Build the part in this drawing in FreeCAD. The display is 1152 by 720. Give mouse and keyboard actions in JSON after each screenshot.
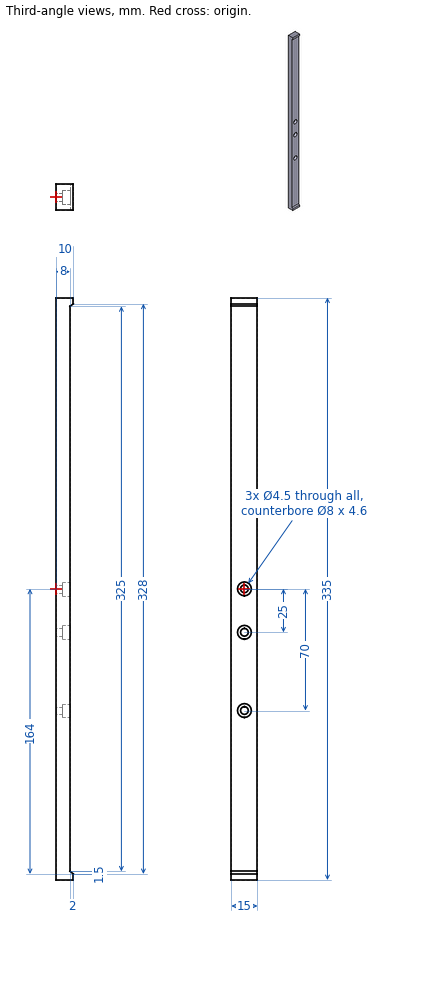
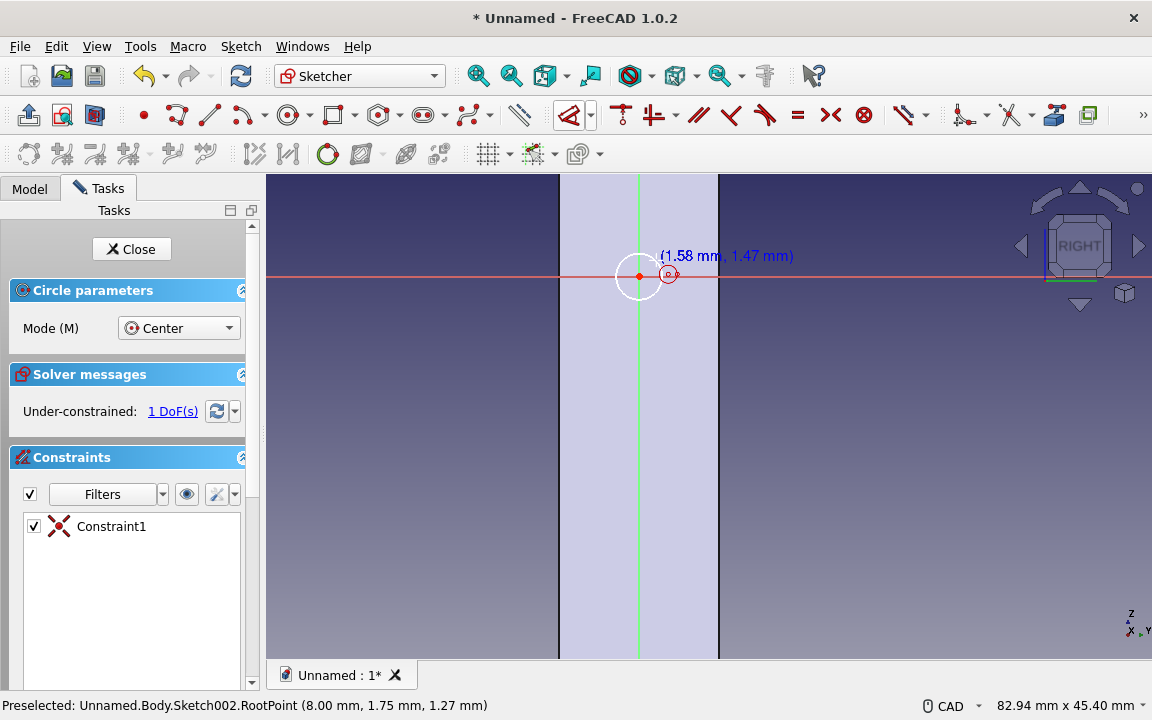
{"action": "scroll", "coordinate": [641, 280], "scroll_direction": "down", "scroll_amount": 5}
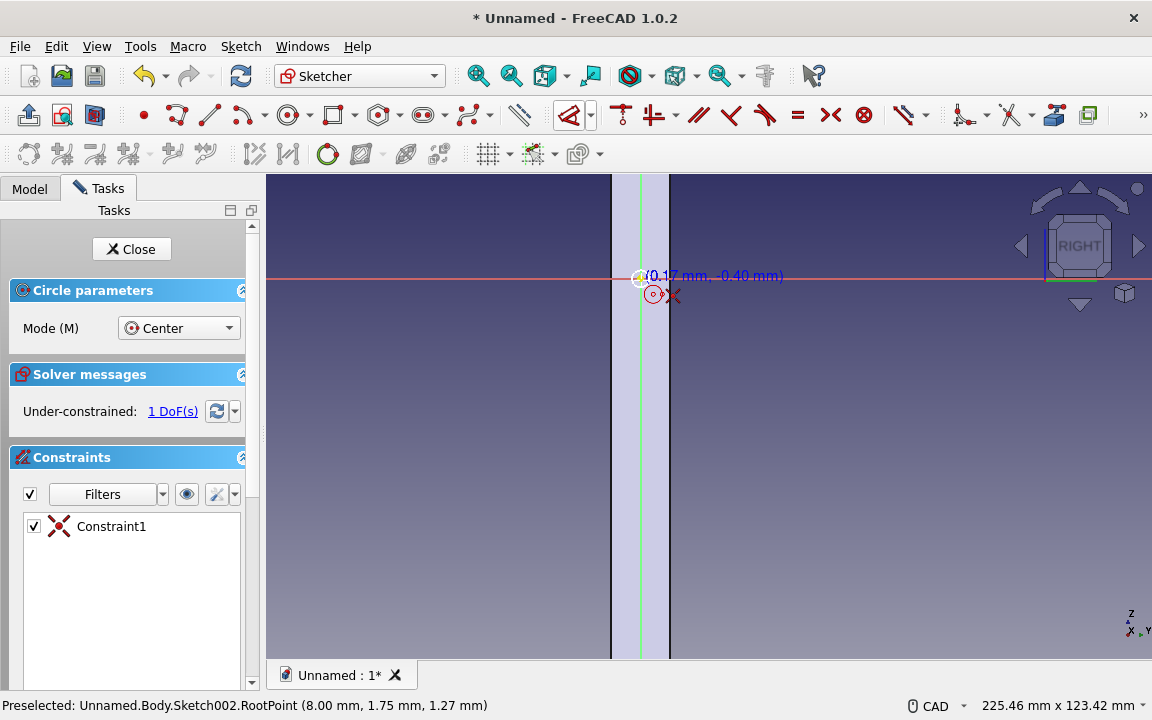
{"action": "scroll", "coordinate": [641, 554], "scroll_direction": "up", "scroll_amount": 5}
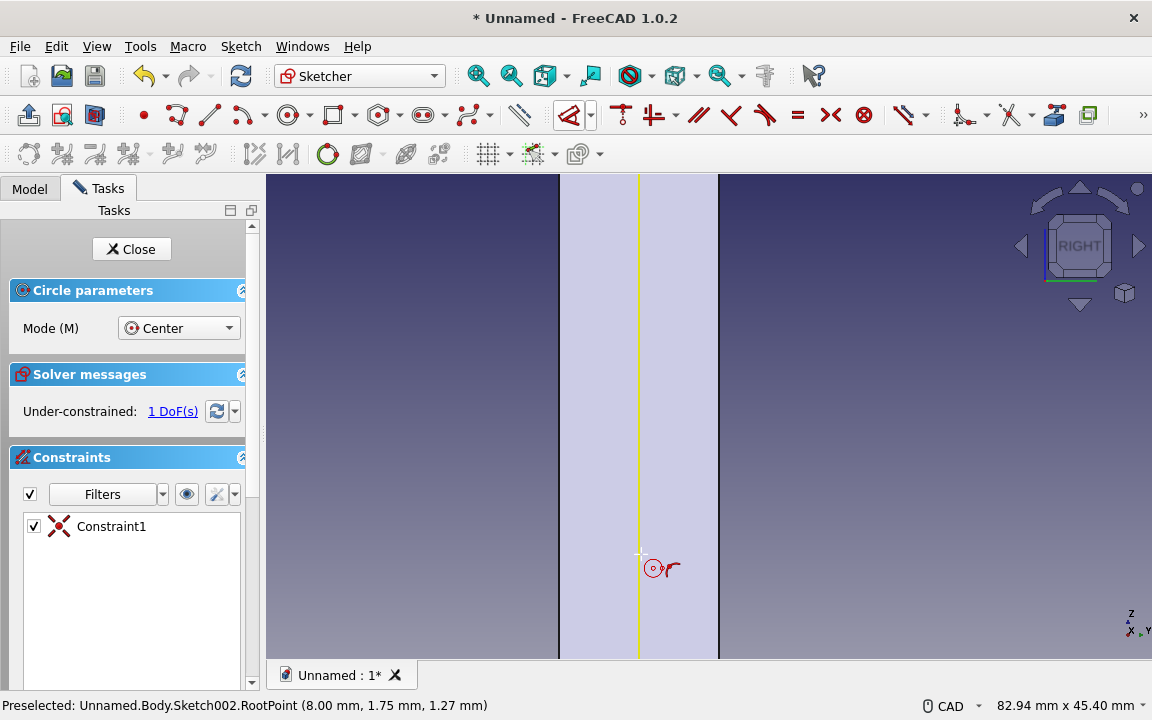
{"action": "left_click", "coordinate": [639, 553]}
{"action": "left_click", "coordinate": [656, 536]}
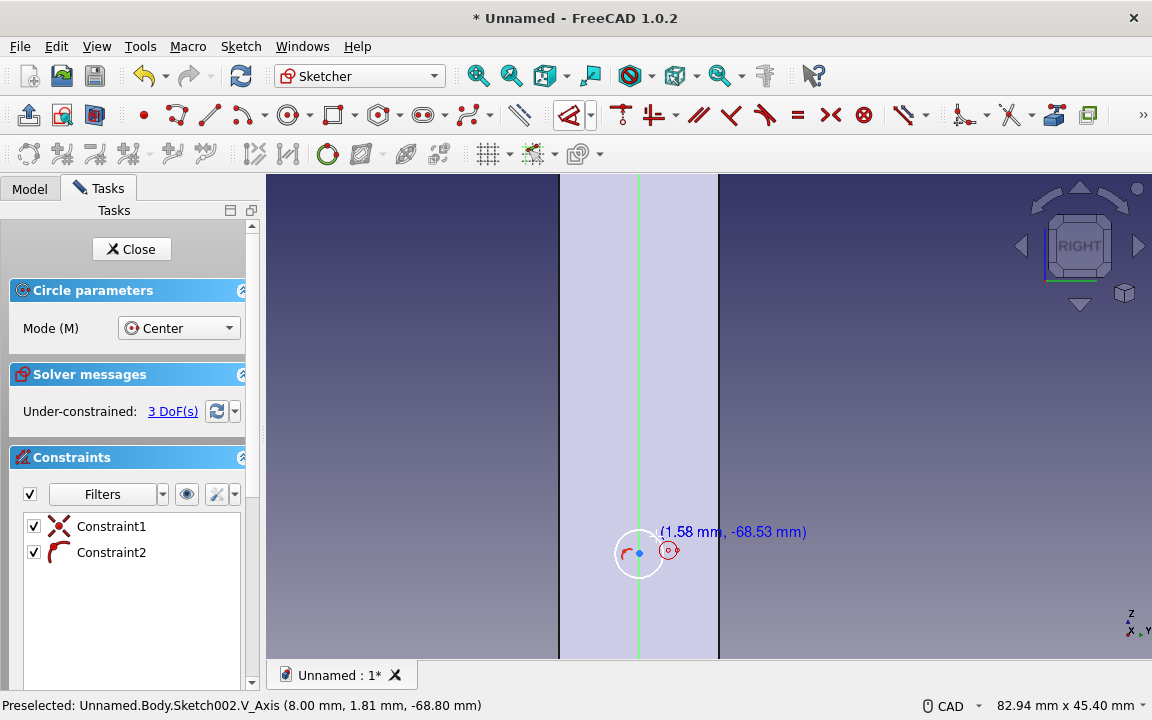
{"action": "scroll", "coordinate": [641, 555], "scroll_direction": "down", "scroll_amount": 5}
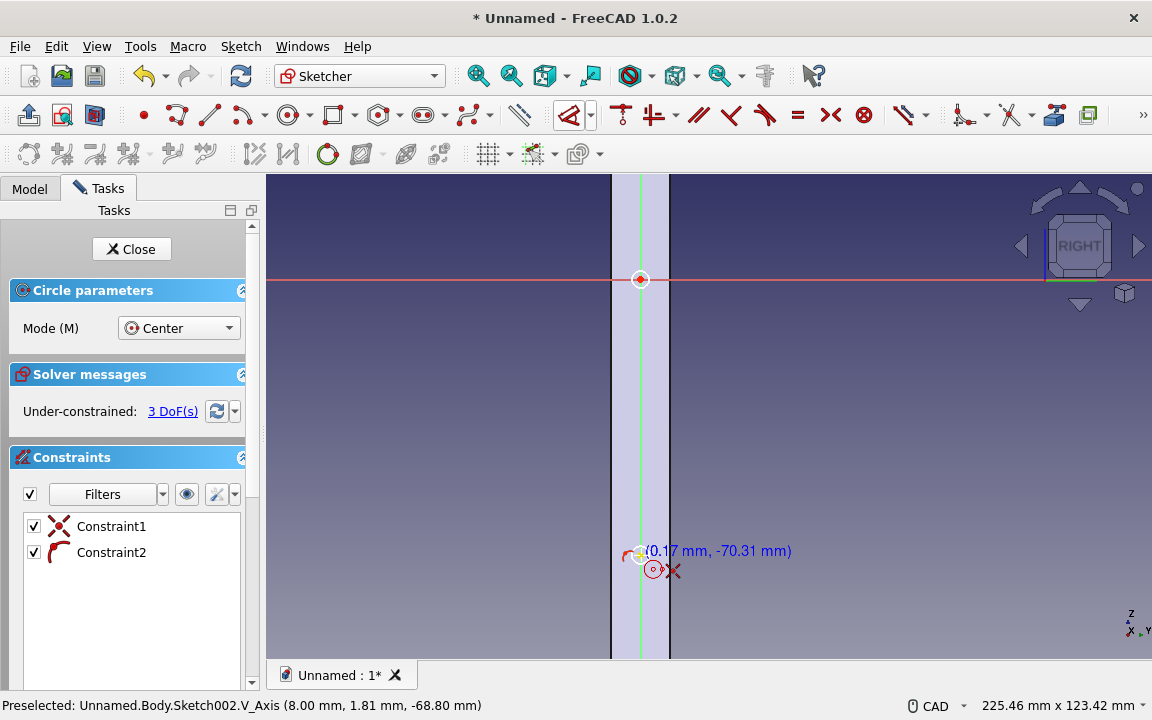
{"action": "scroll", "coordinate": [641, 378], "scroll_direction": "up", "scroll_amount": 5}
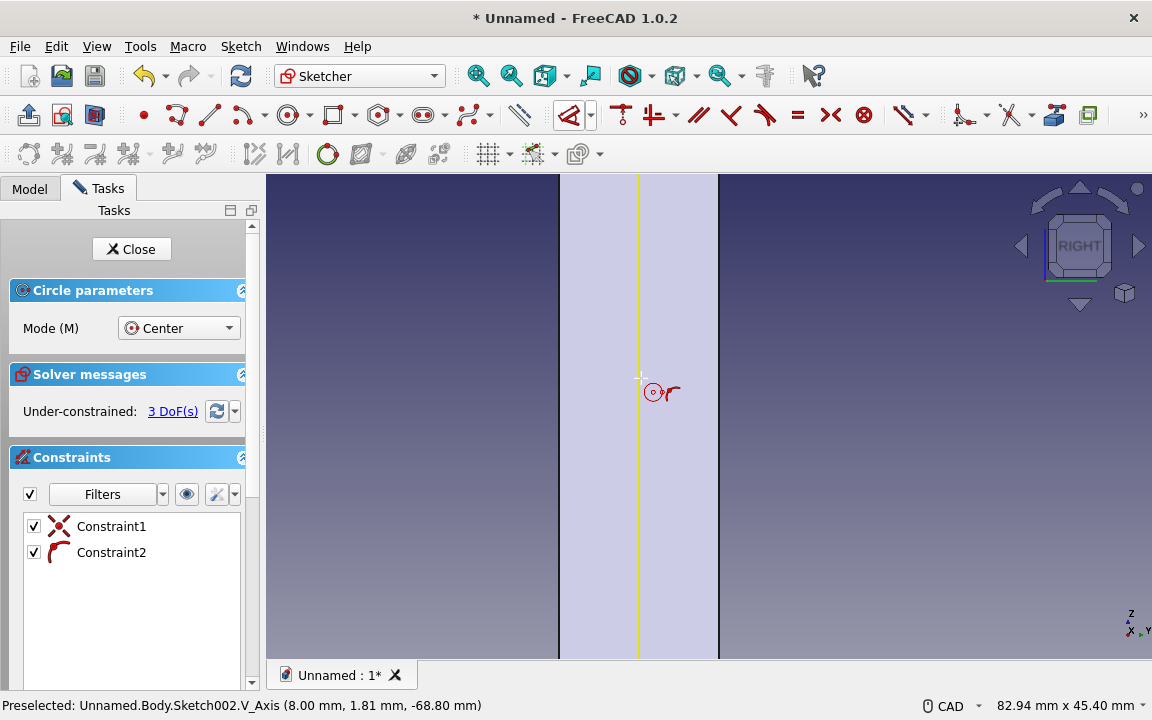
{"action": "left_click", "coordinate": [639, 377]}
{"action": "left_click", "coordinate": [656, 360]}
{"action": "key", "text": "Escape"}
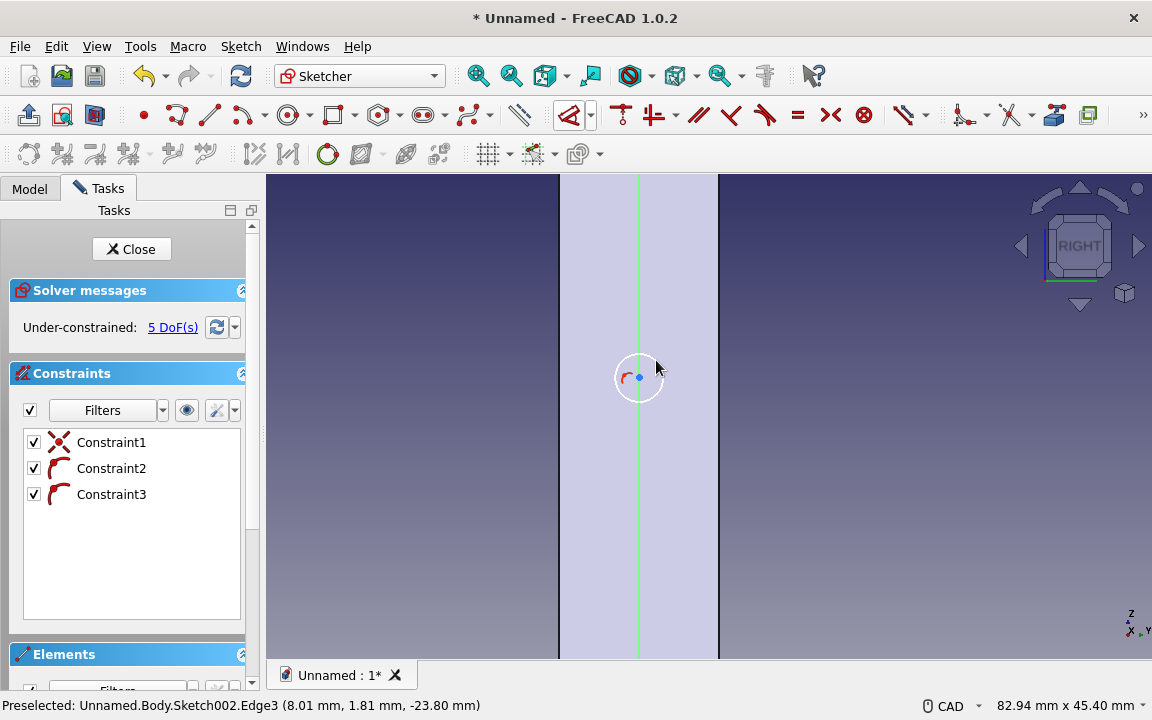
{"action": "scroll", "coordinate": [641, 377], "scroll_direction": "down", "scroll_amount": 5}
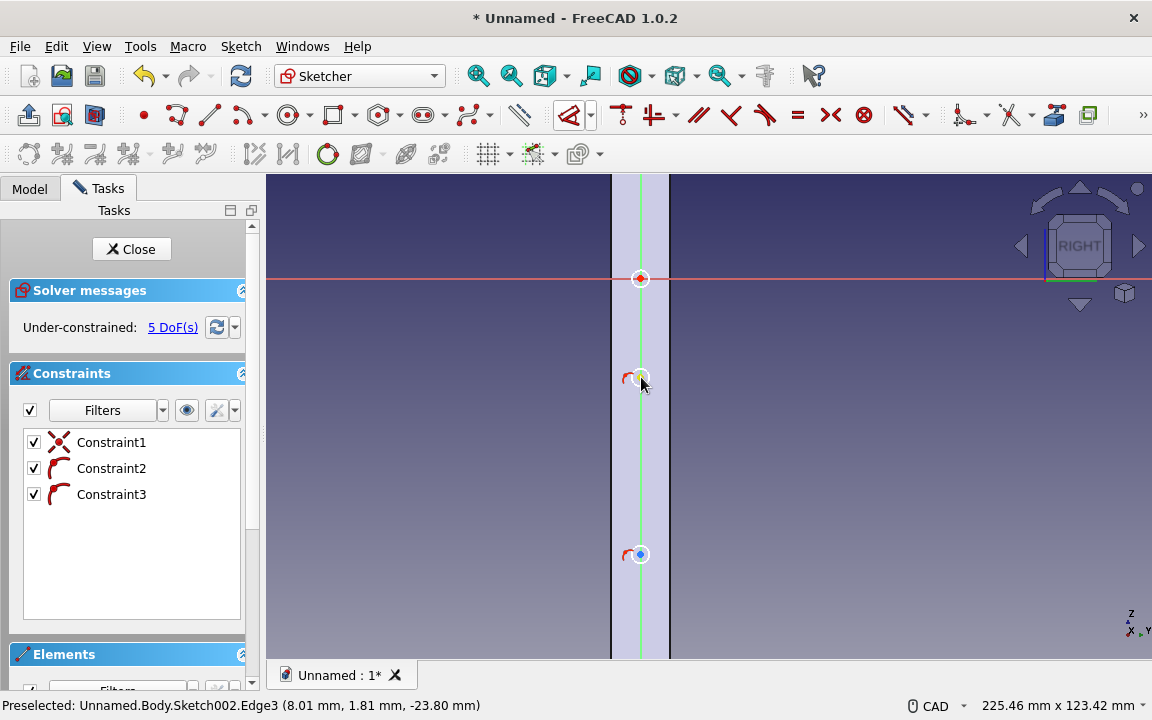
{"action": "scroll", "coordinate": [647, 273], "scroll_direction": "up", "scroll_amount": 5}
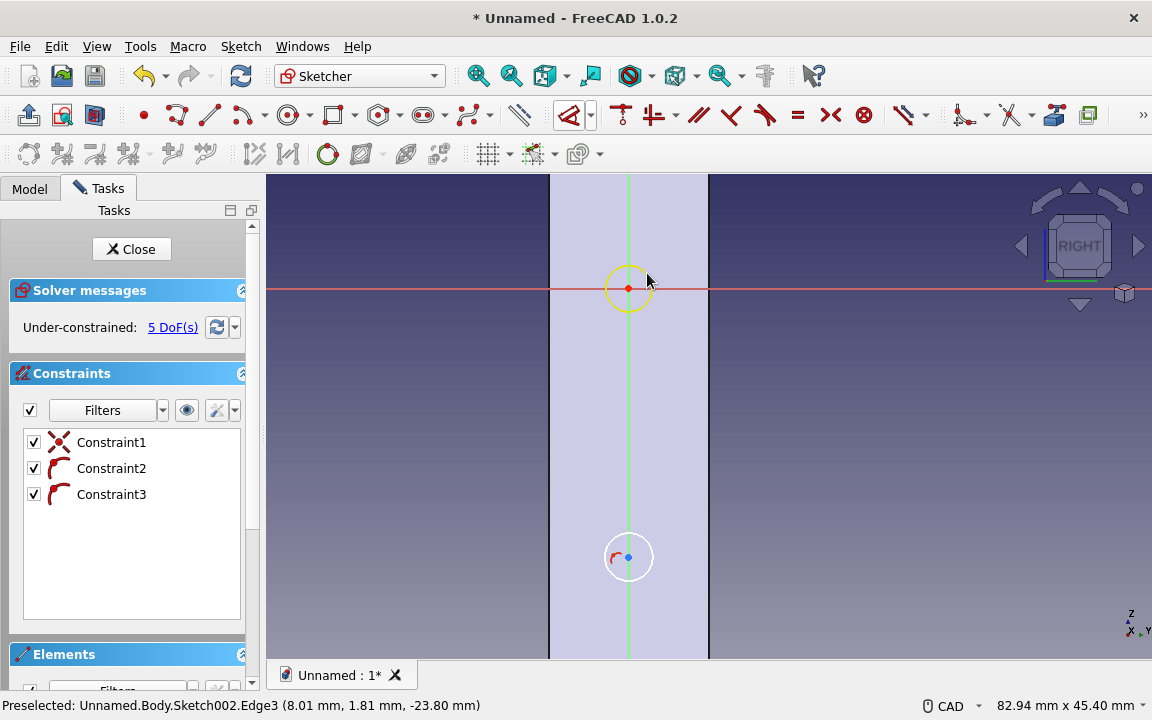
{"action": "left_click", "coordinate": [645, 272]}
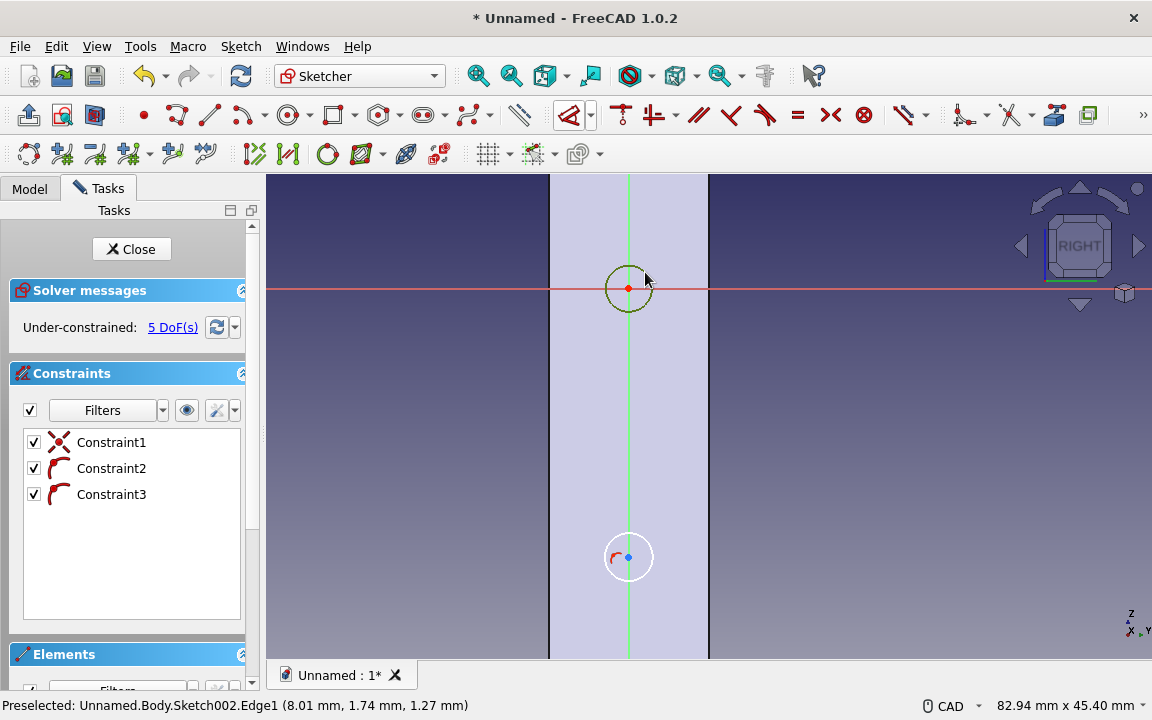
{"action": "scroll", "coordinate": [647, 273], "scroll_direction": "down", "scroll_amount": 5}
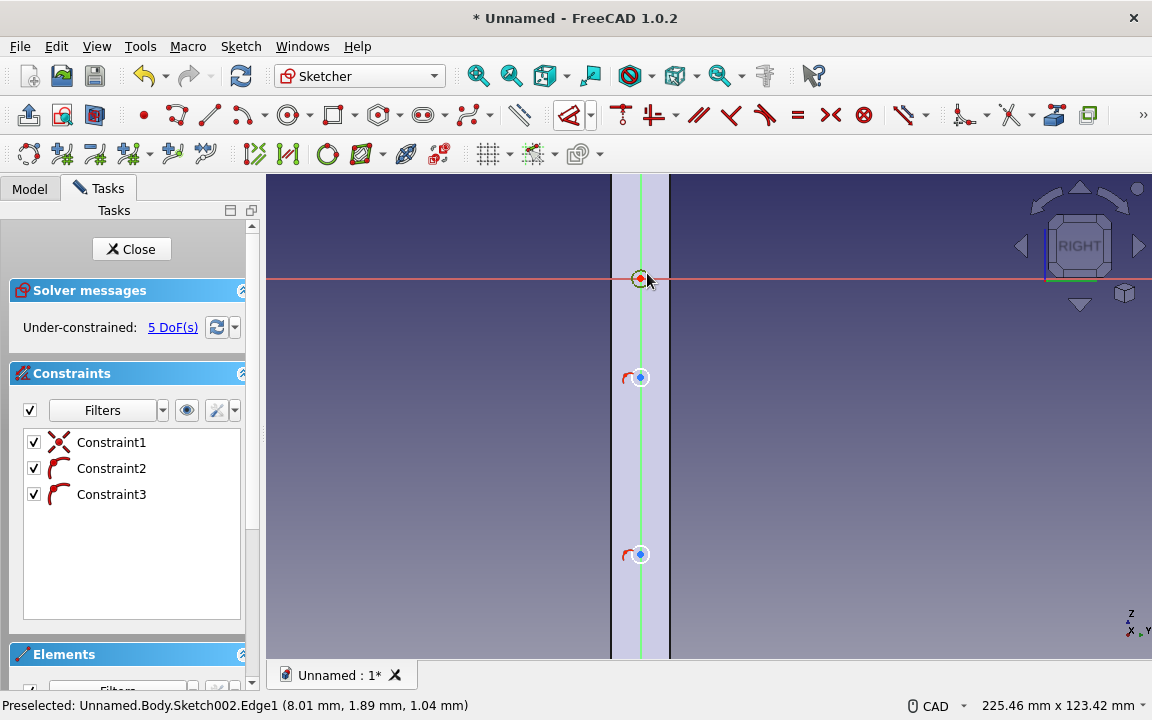
{"action": "scroll", "coordinate": [647, 548], "scroll_direction": "up", "scroll_amount": 5}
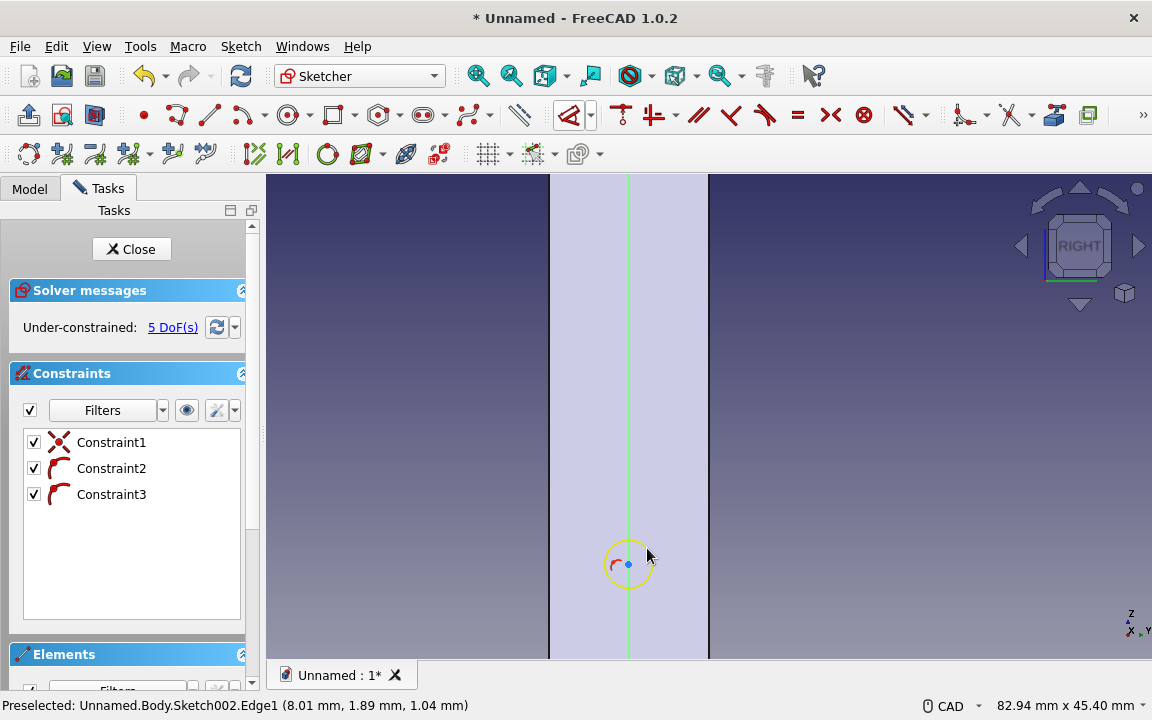
{"action": "left_click", "coordinate": [646, 547]}